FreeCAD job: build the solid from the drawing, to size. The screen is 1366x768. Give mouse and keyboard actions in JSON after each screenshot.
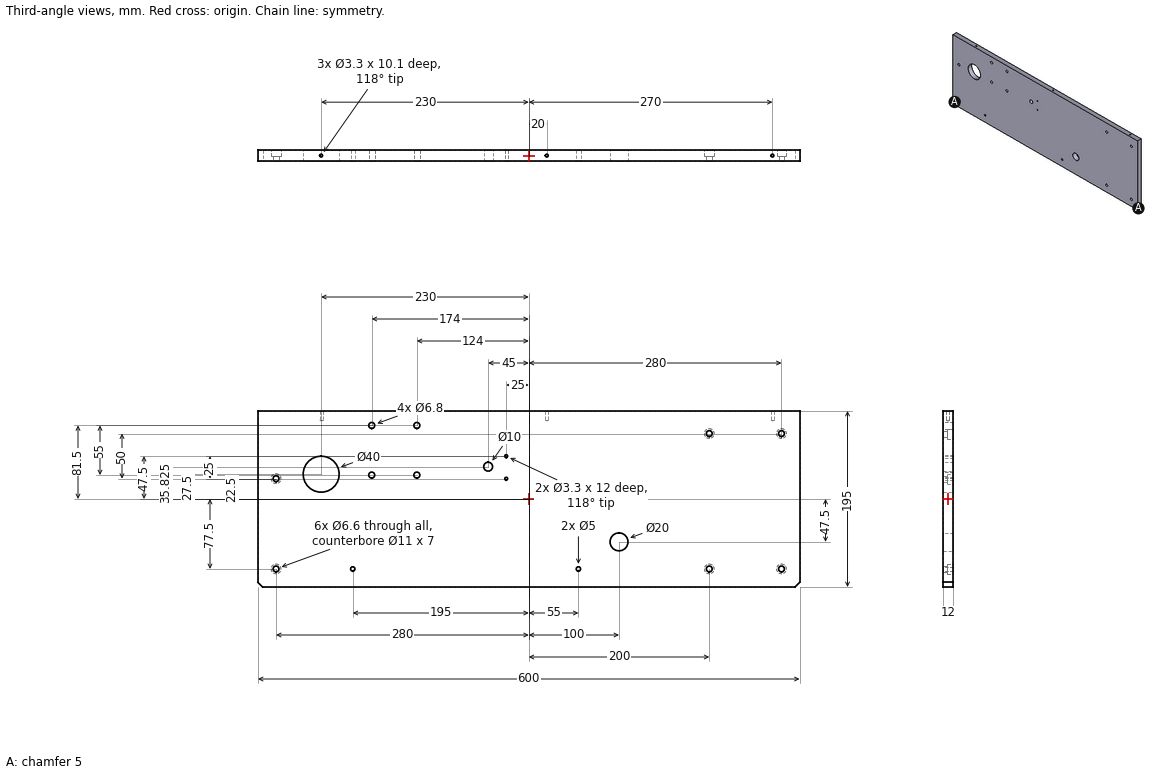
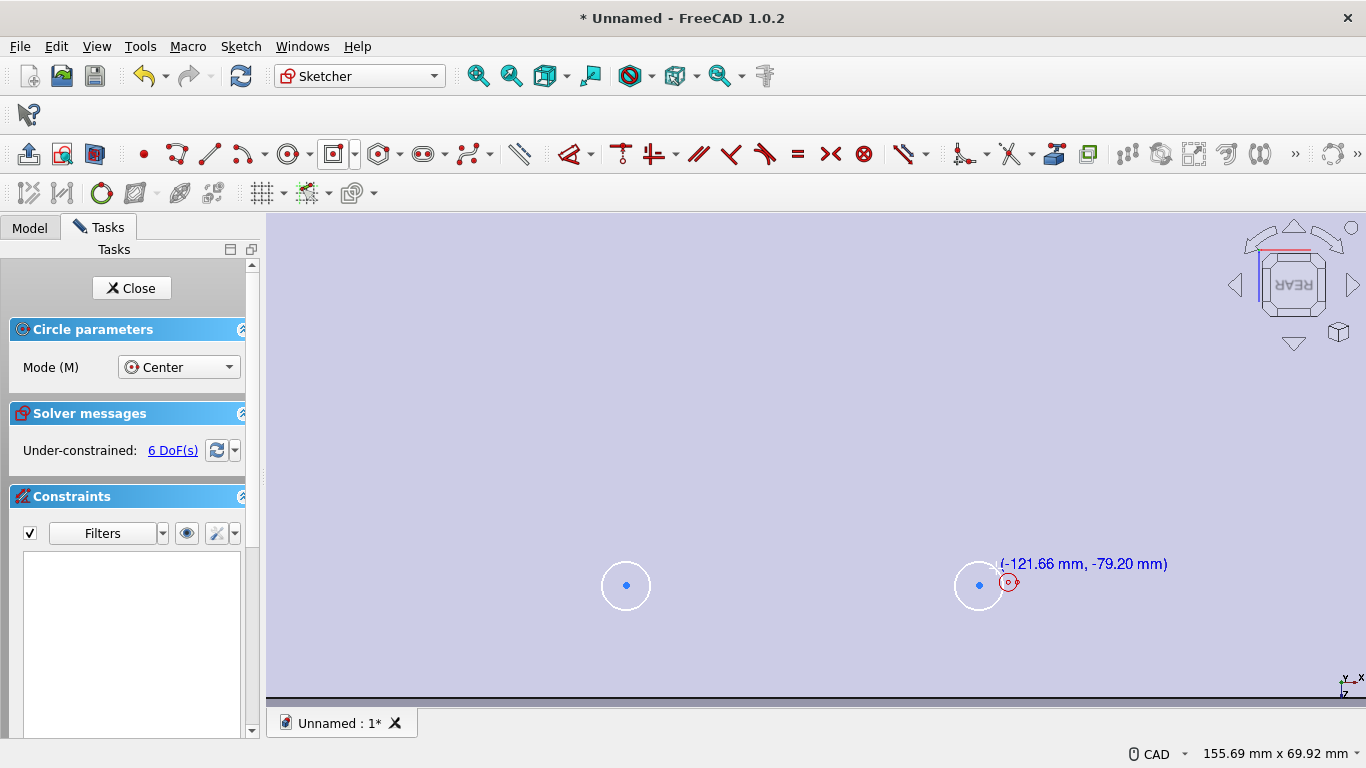
{"action": "scroll", "coordinate": [635, 600], "scroll_direction": "down", "scroll_amount": 2}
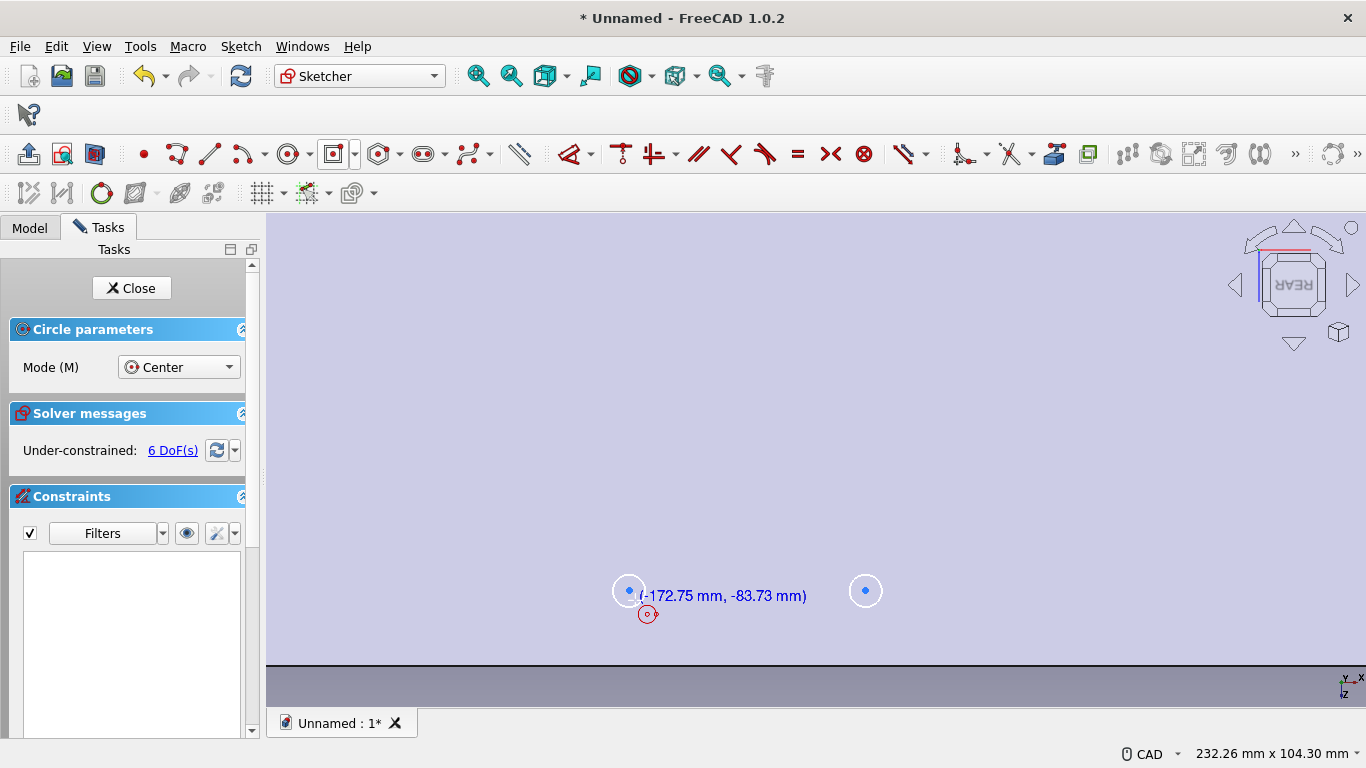
{"action": "scroll", "coordinate": [866, 330], "scroll_direction": "up", "scroll_amount": 2}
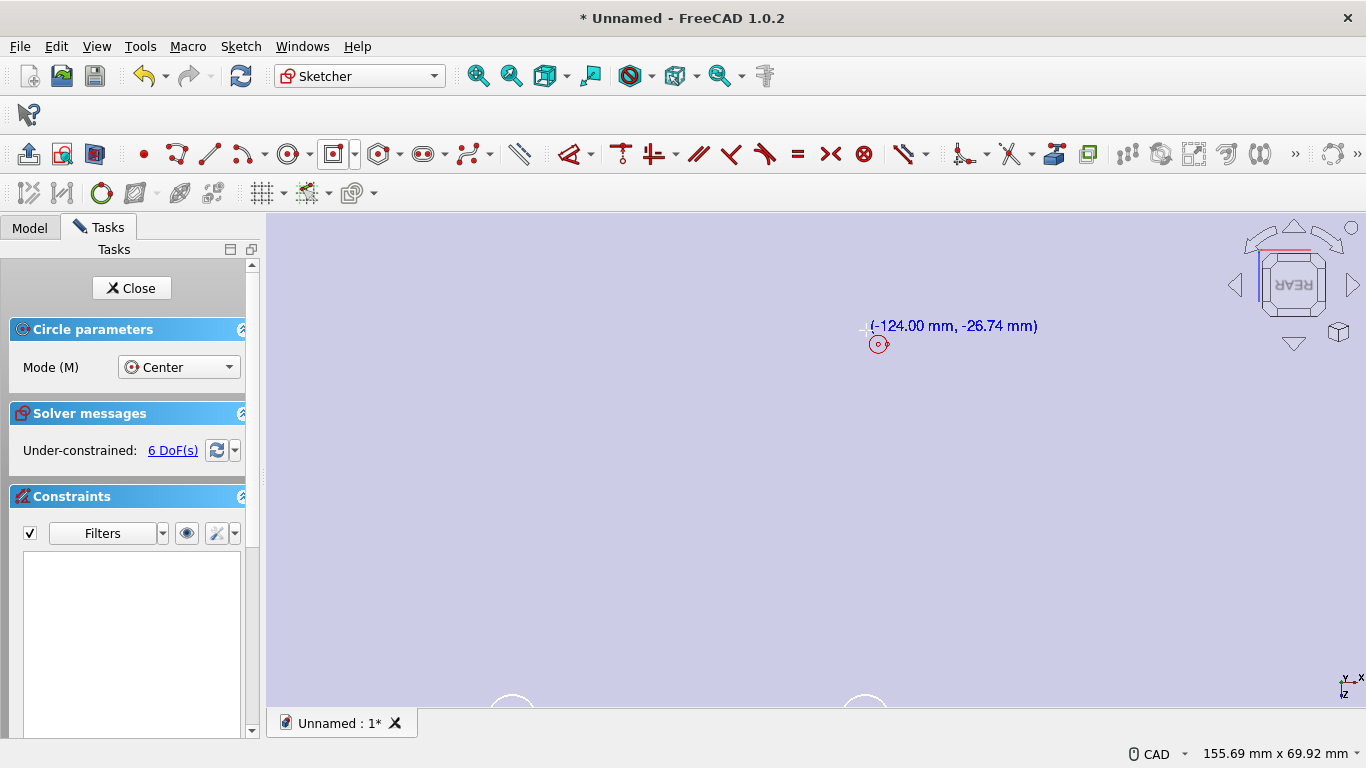
{"action": "left_click", "coordinate": [866, 330]}
{"action": "left_click", "coordinate": [883, 313]}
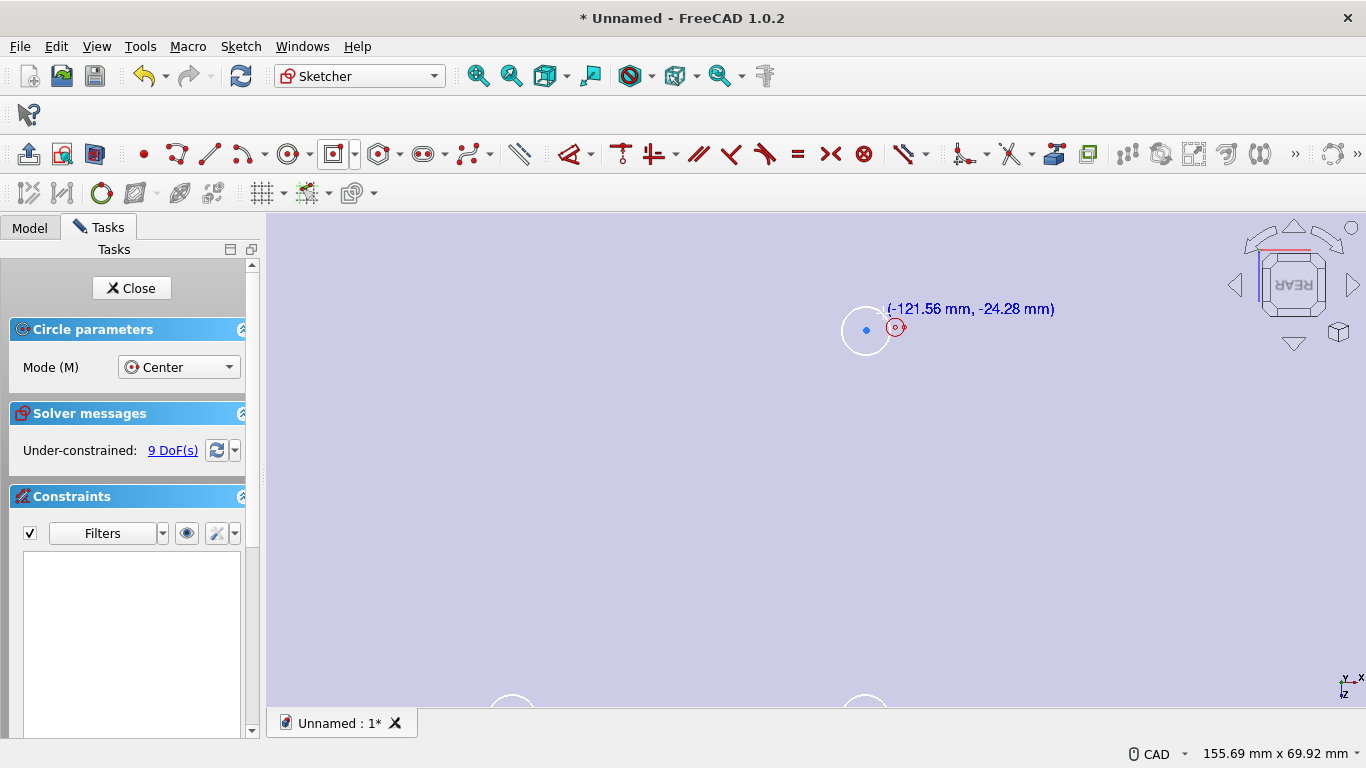
{"action": "left_click", "coordinate": [512, 330]}
{"action": "left_click", "coordinate": [529, 313]}
{"action": "key", "text": "Escape"}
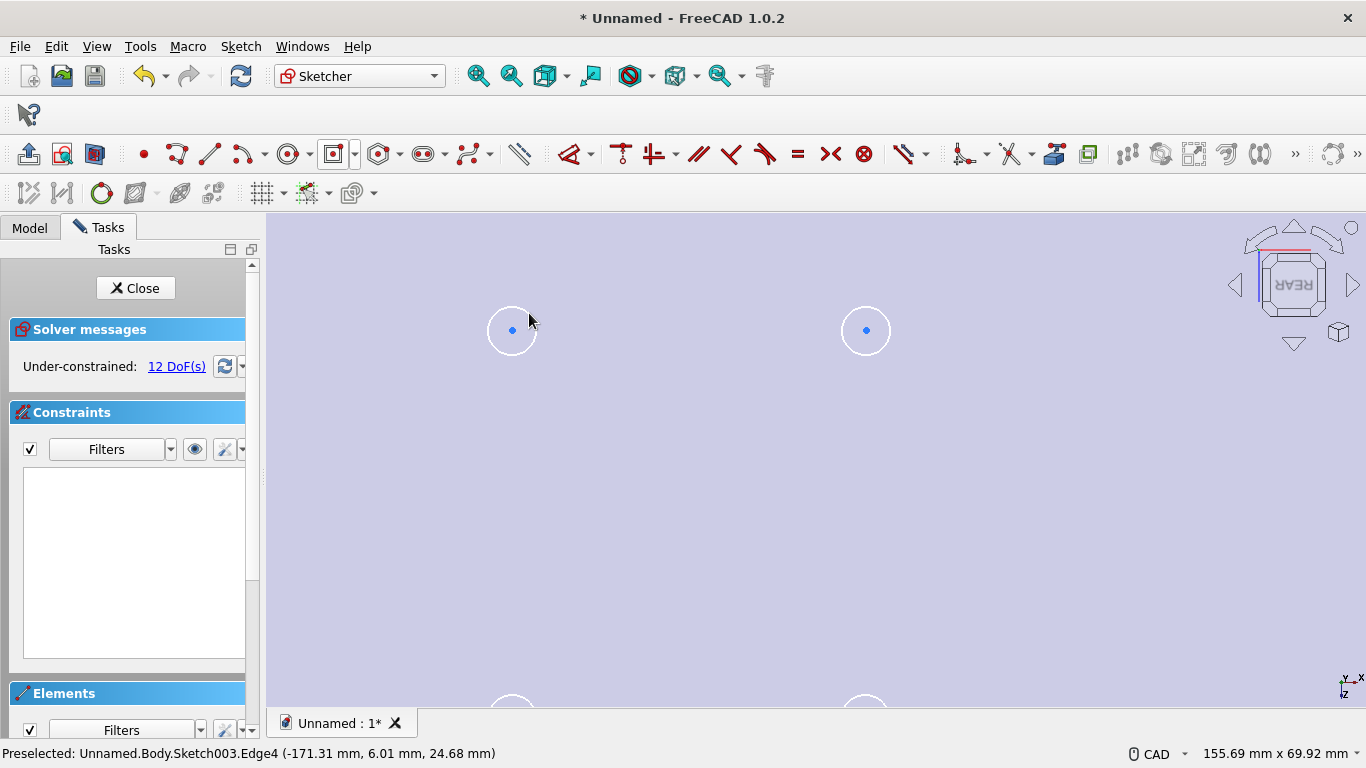
{"action": "scroll", "coordinate": [866, 330], "scroll_direction": "down", "scroll_amount": 2}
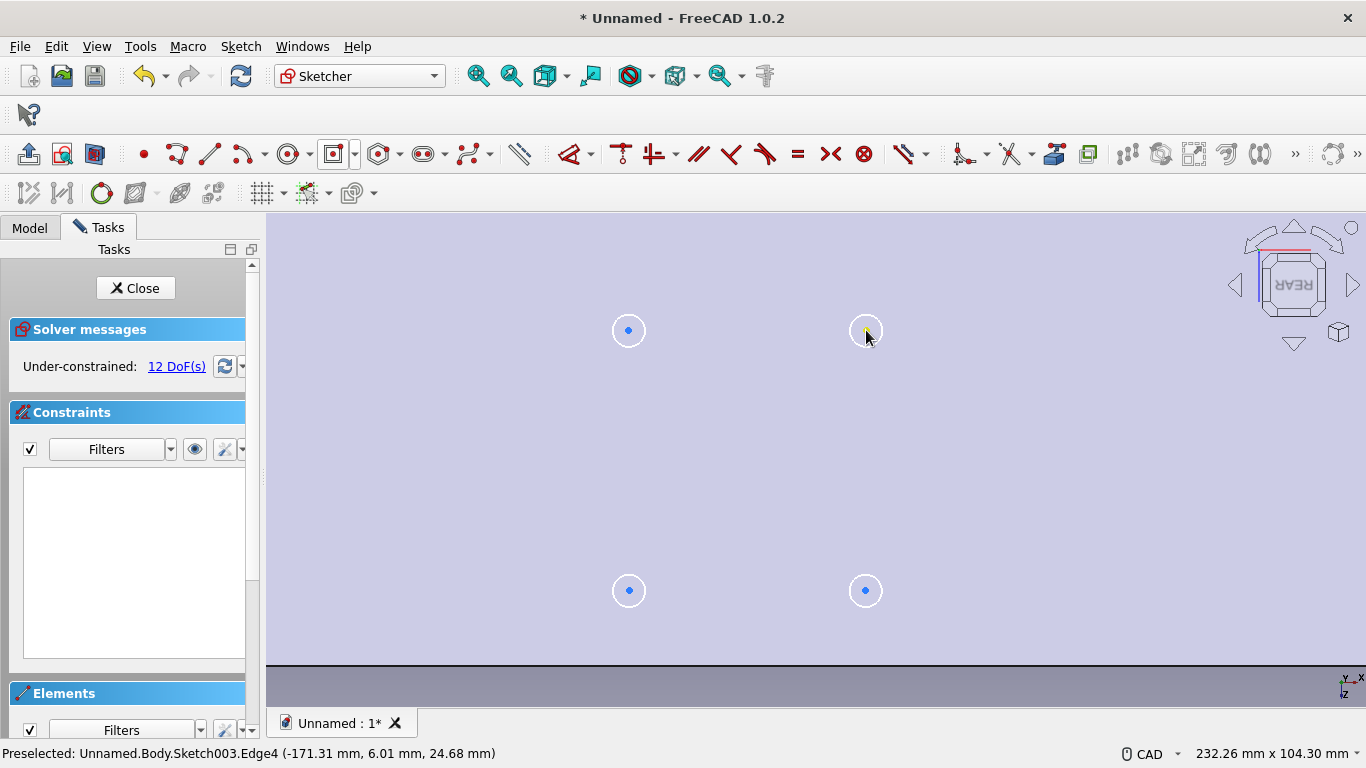
{"action": "left_click", "coordinate": [640, 579]}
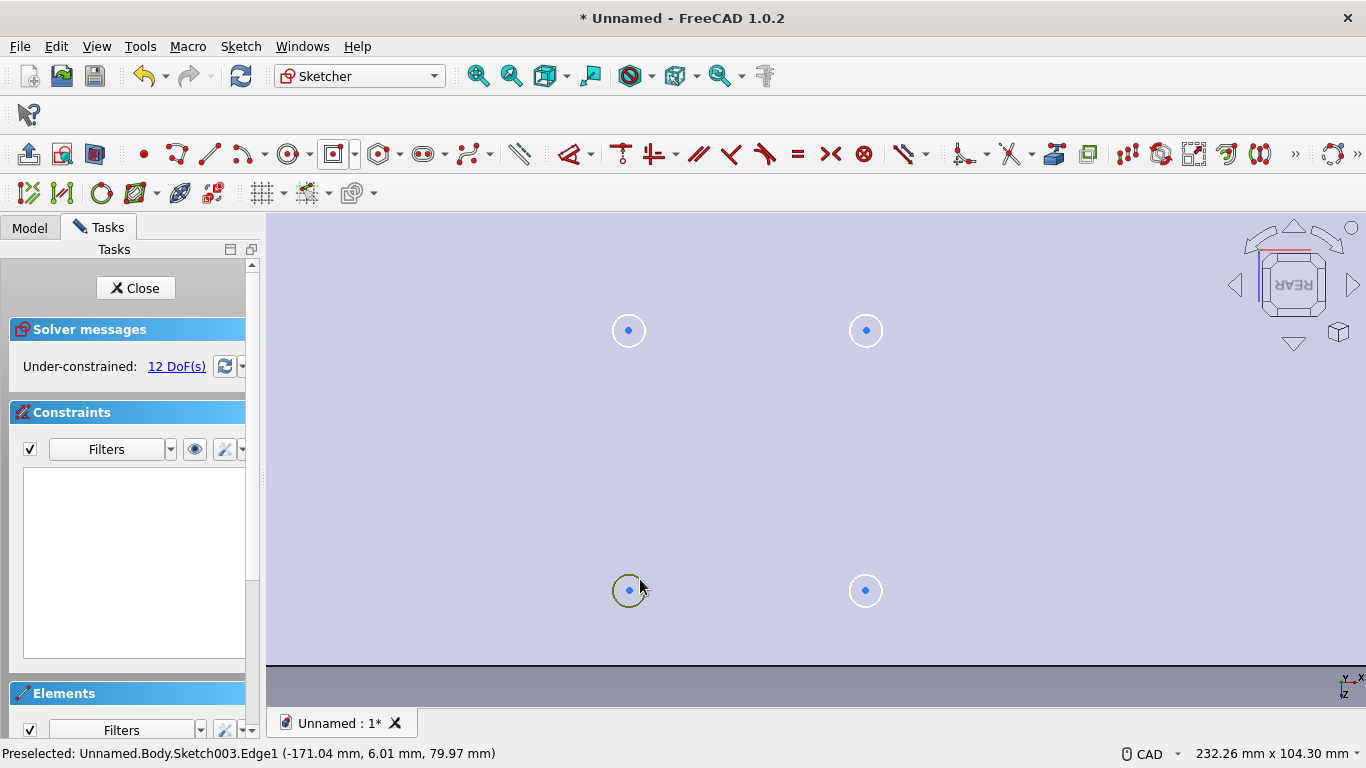
{"action": "left_click", "coordinate": [877, 579]}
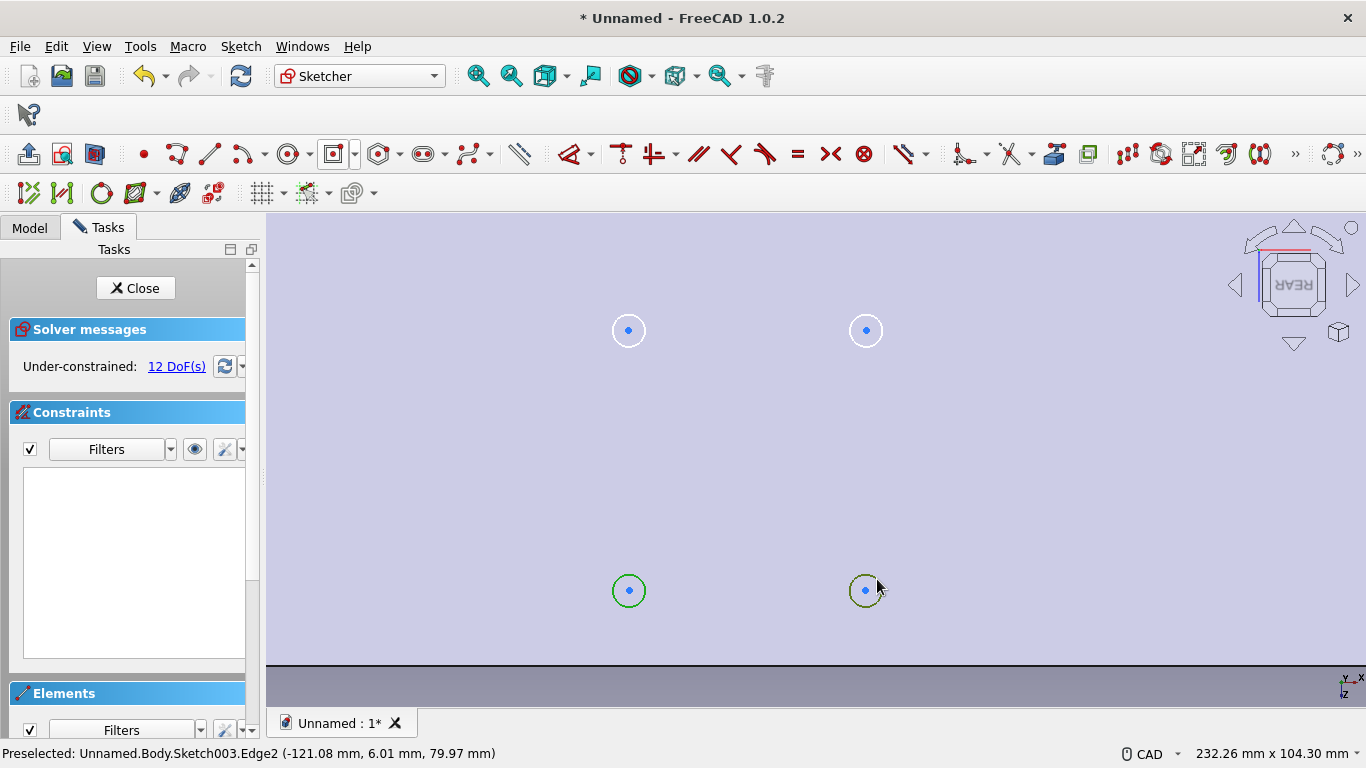
{"action": "left_click", "coordinate": [878, 319]}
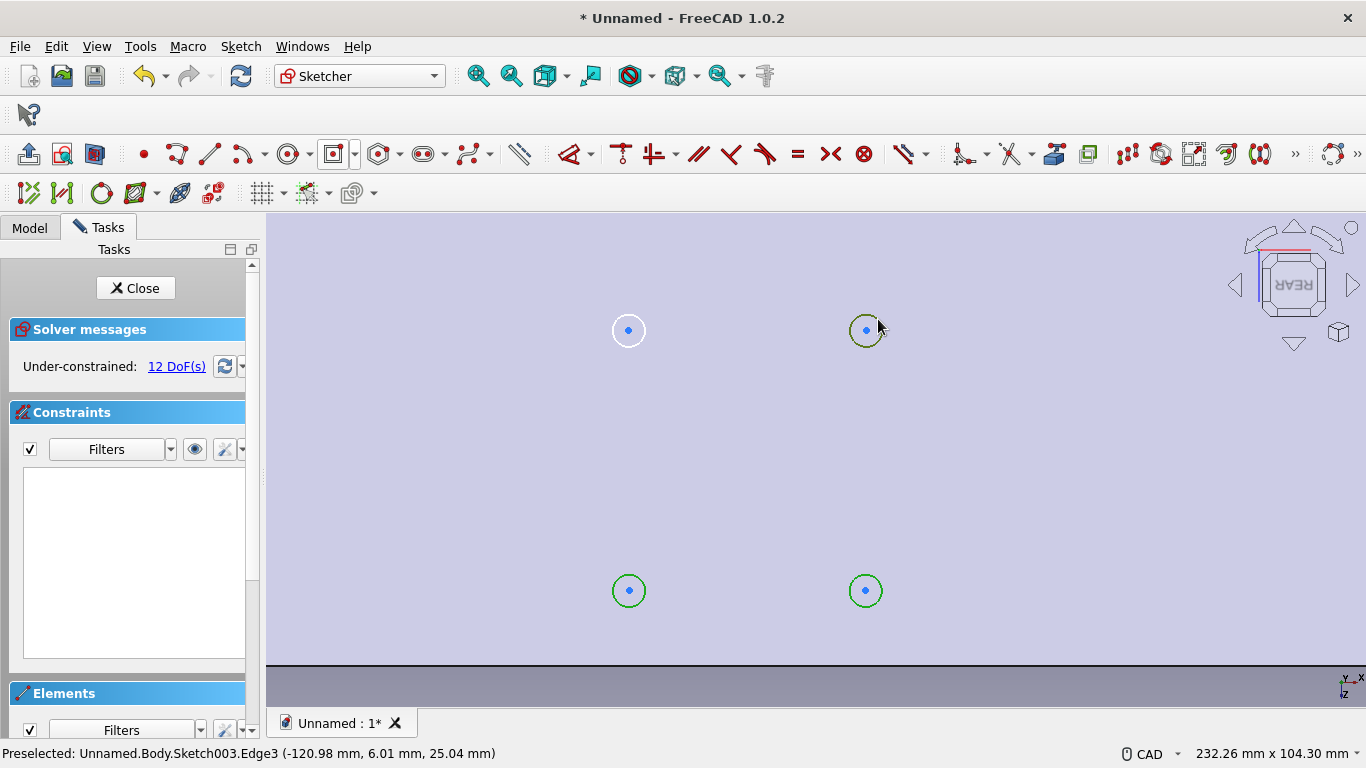
{"action": "left_click", "coordinate": [640, 319]}